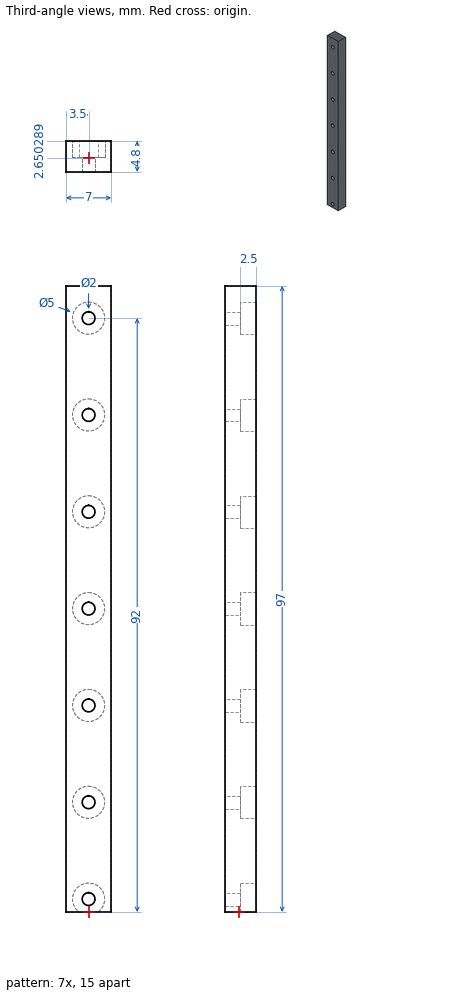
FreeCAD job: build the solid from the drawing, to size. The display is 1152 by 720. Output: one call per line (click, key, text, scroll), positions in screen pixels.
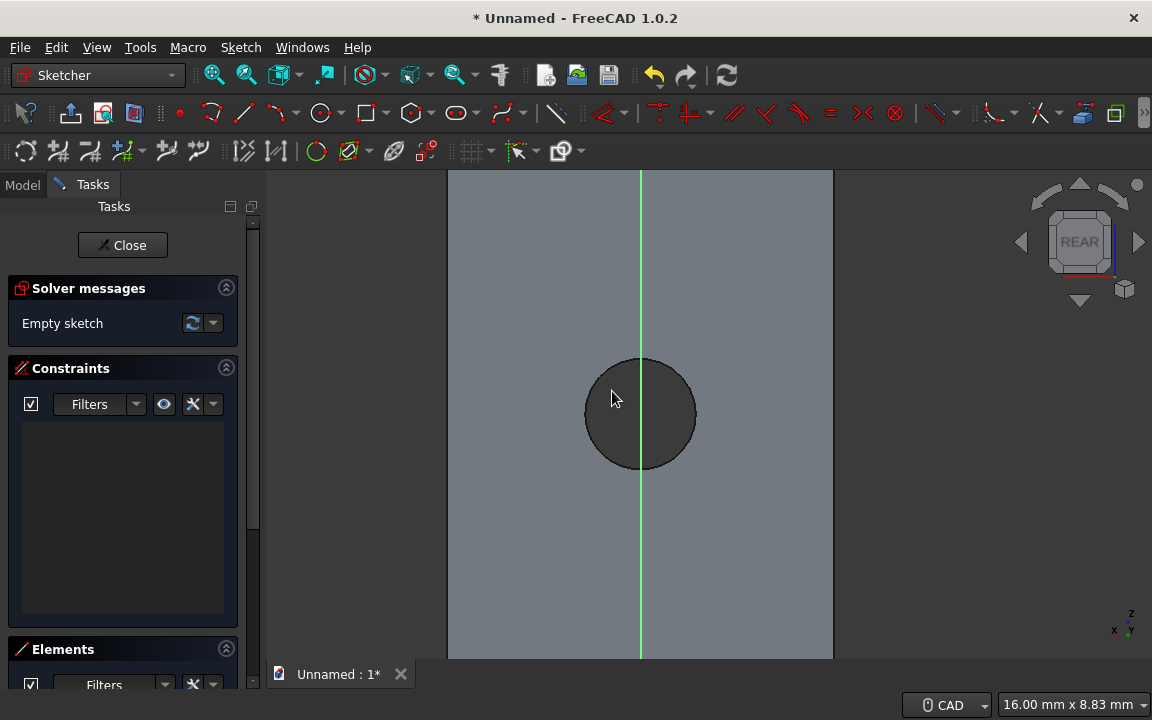
click(322, 114)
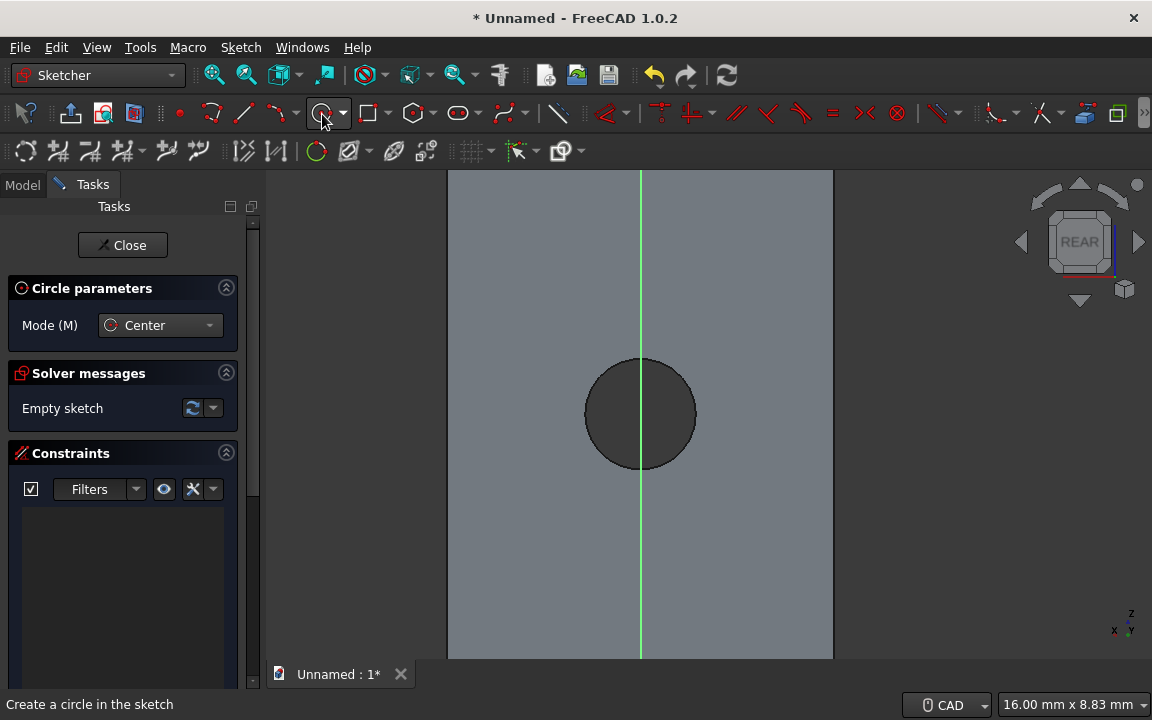
click(641, 414)
move(738, 316)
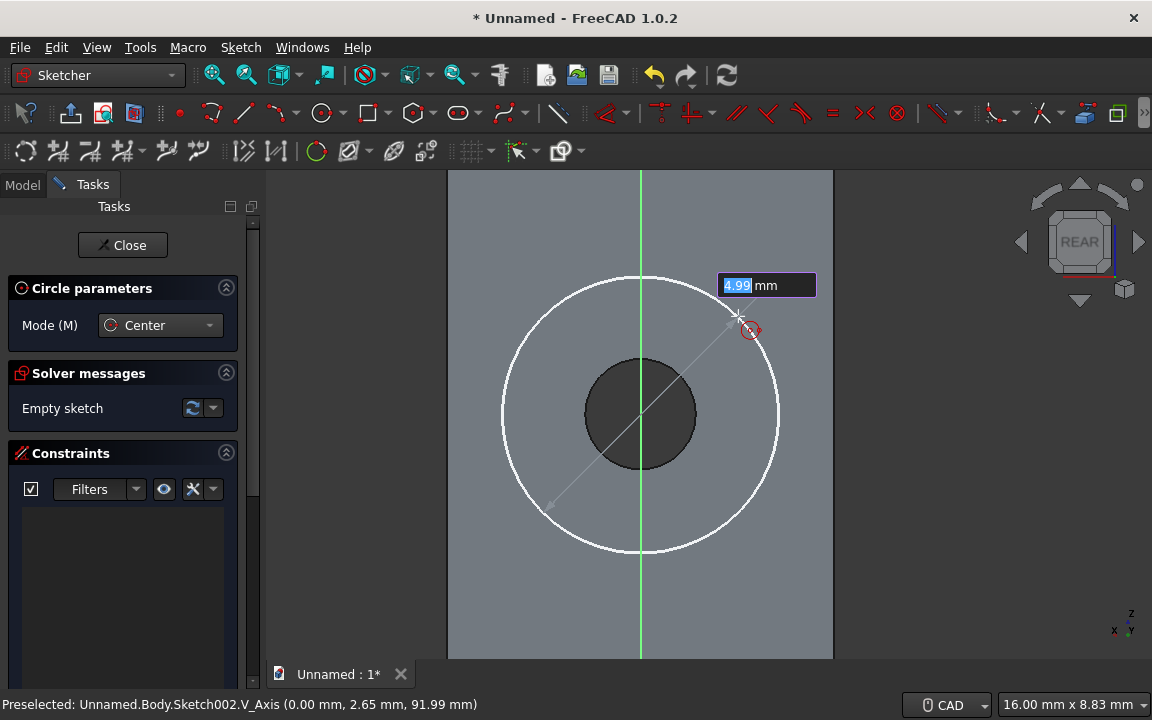
text(5)
key(Return)
key(Escape)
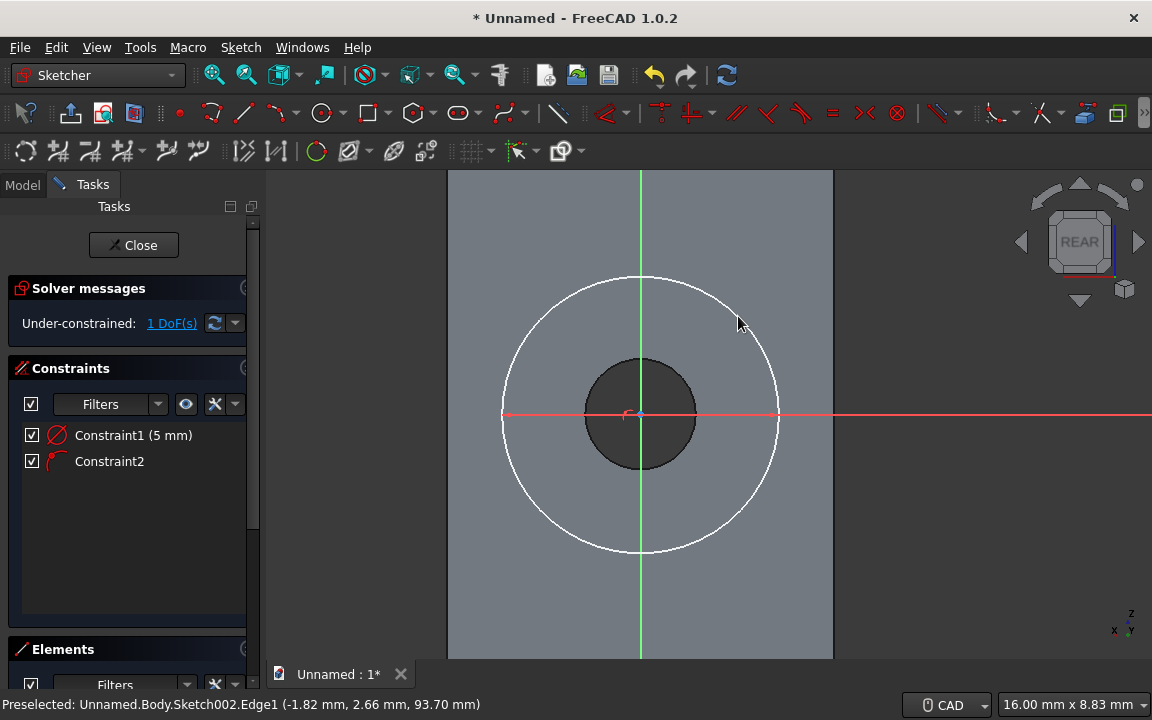
key(d)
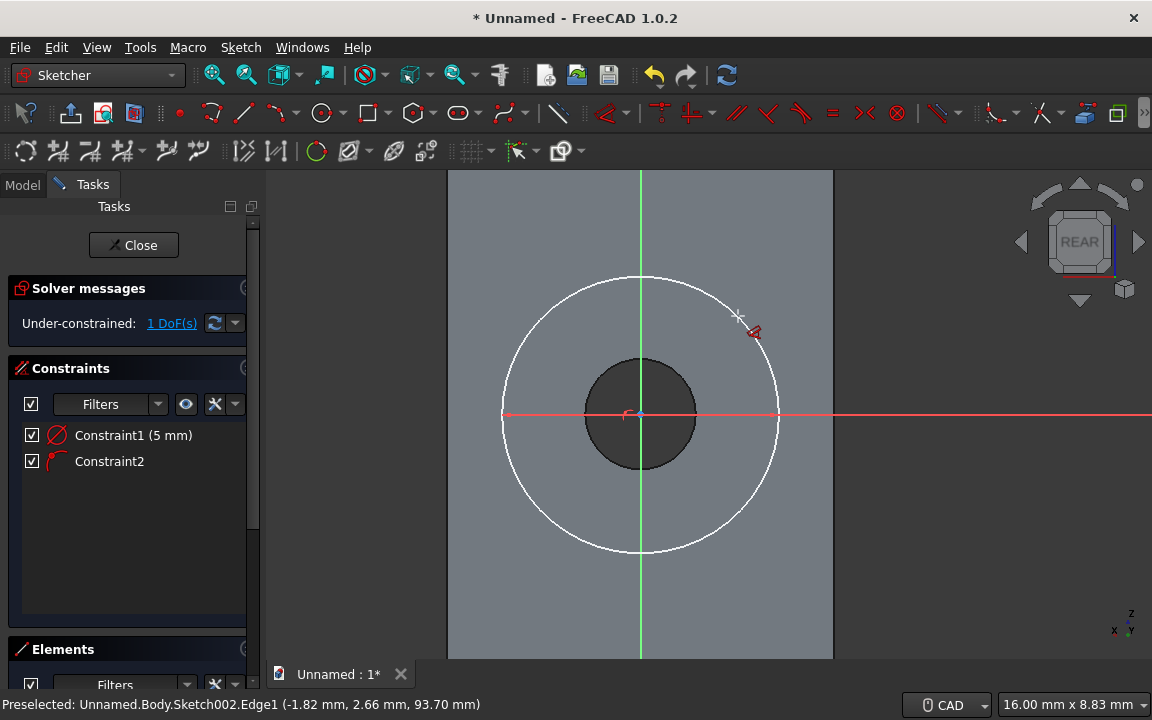
click(641, 415)
click(675, 523)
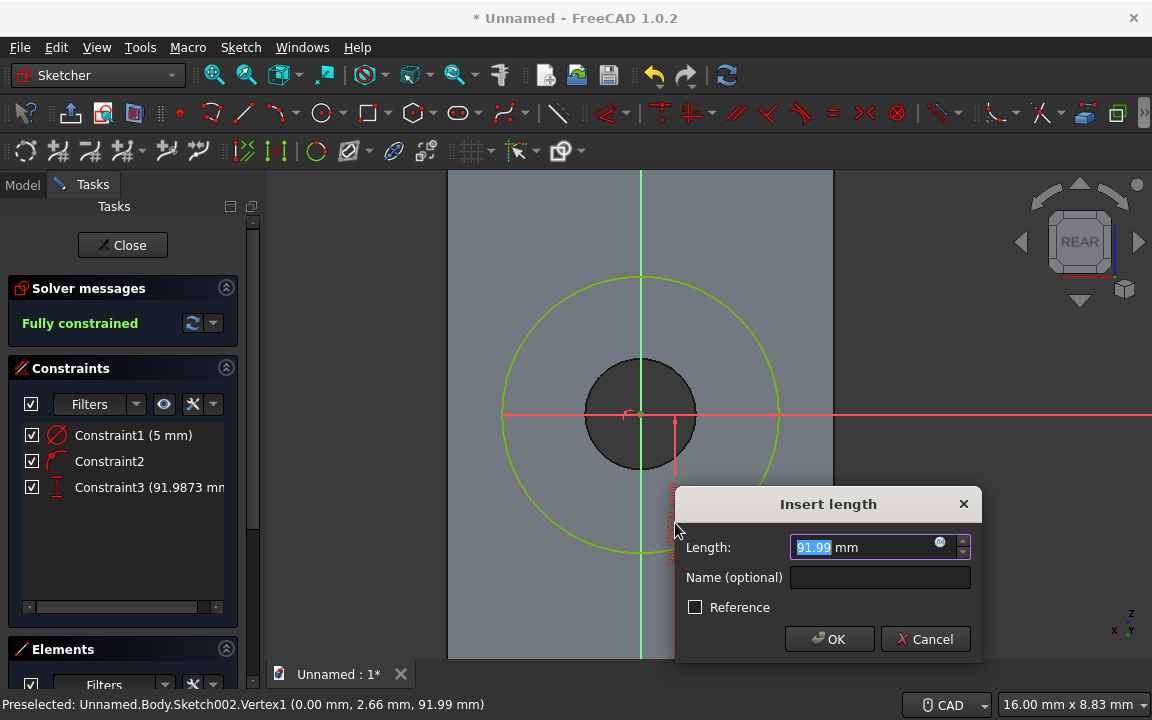
text(92)
key(Return)
key(Escape)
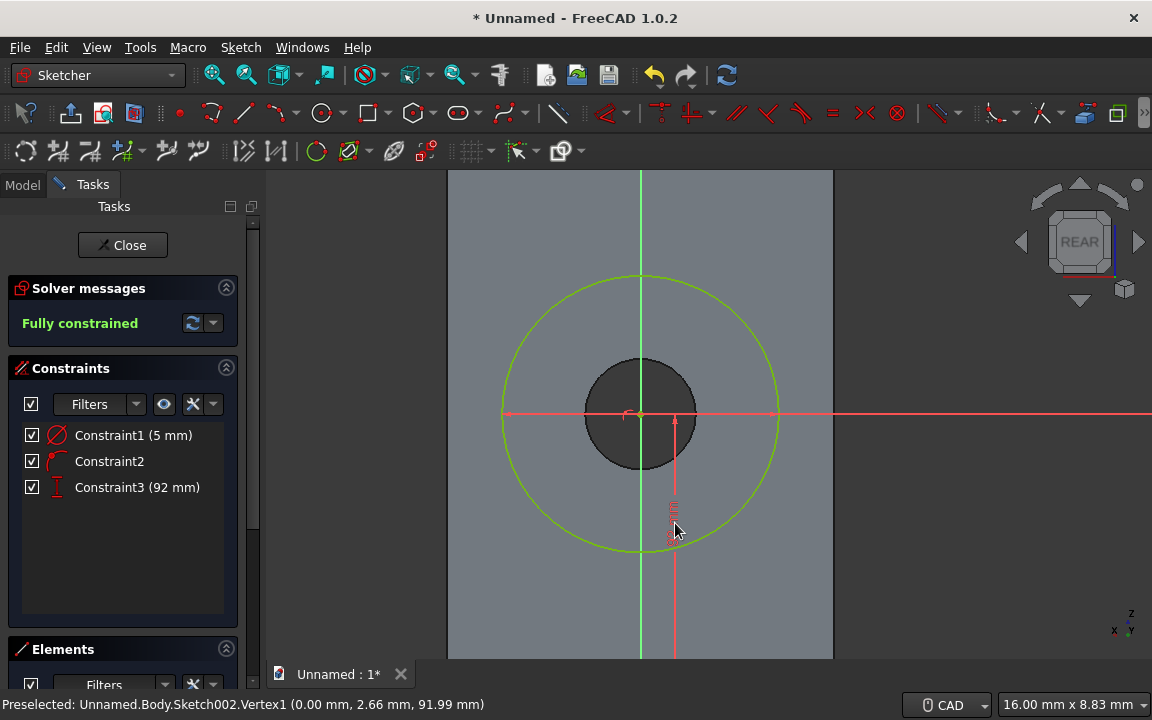
click(123, 245)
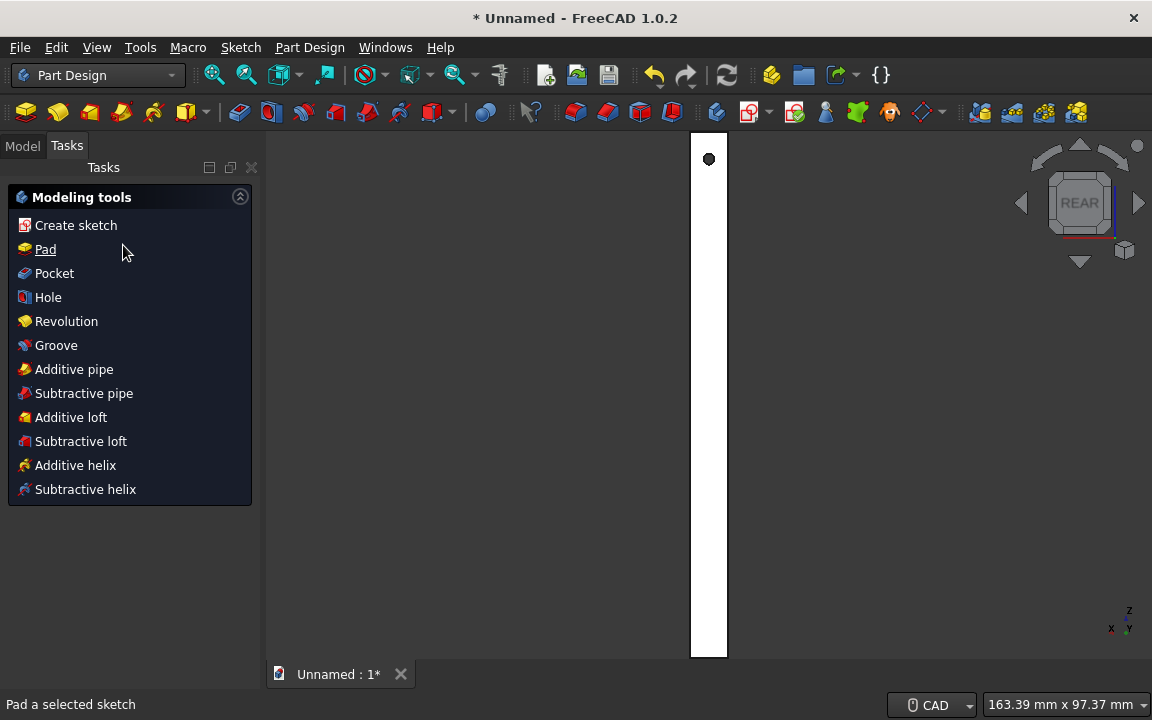
click(240, 112)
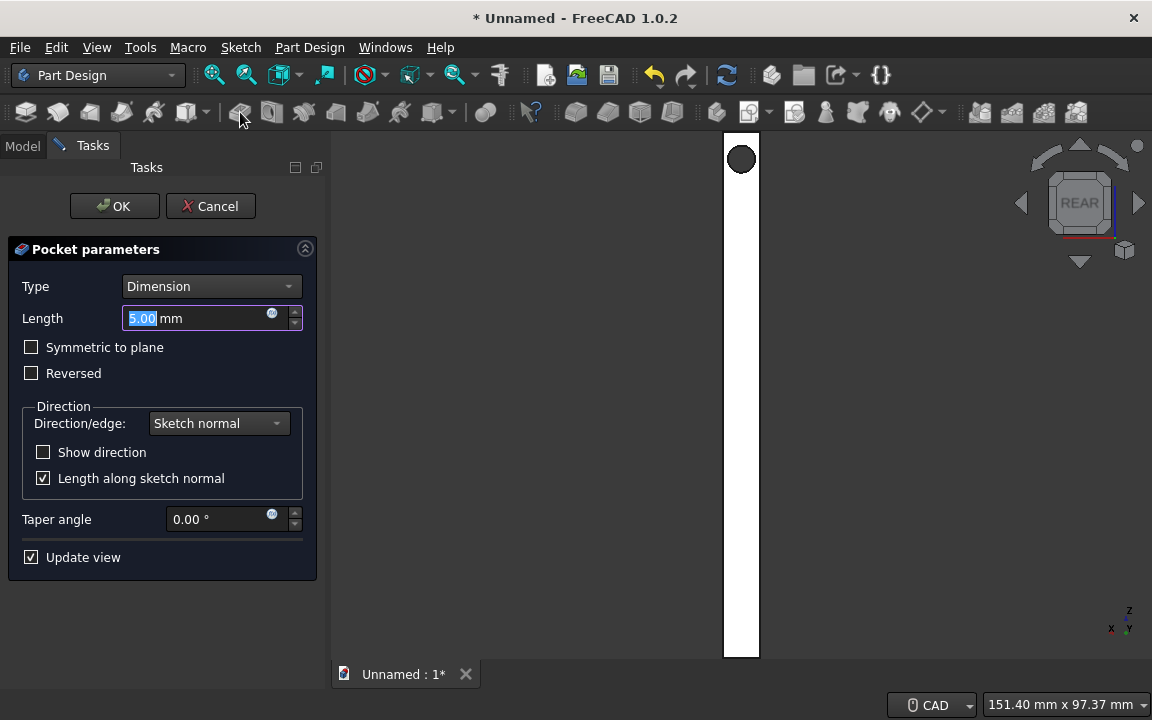
text(2.5)
key(Tab)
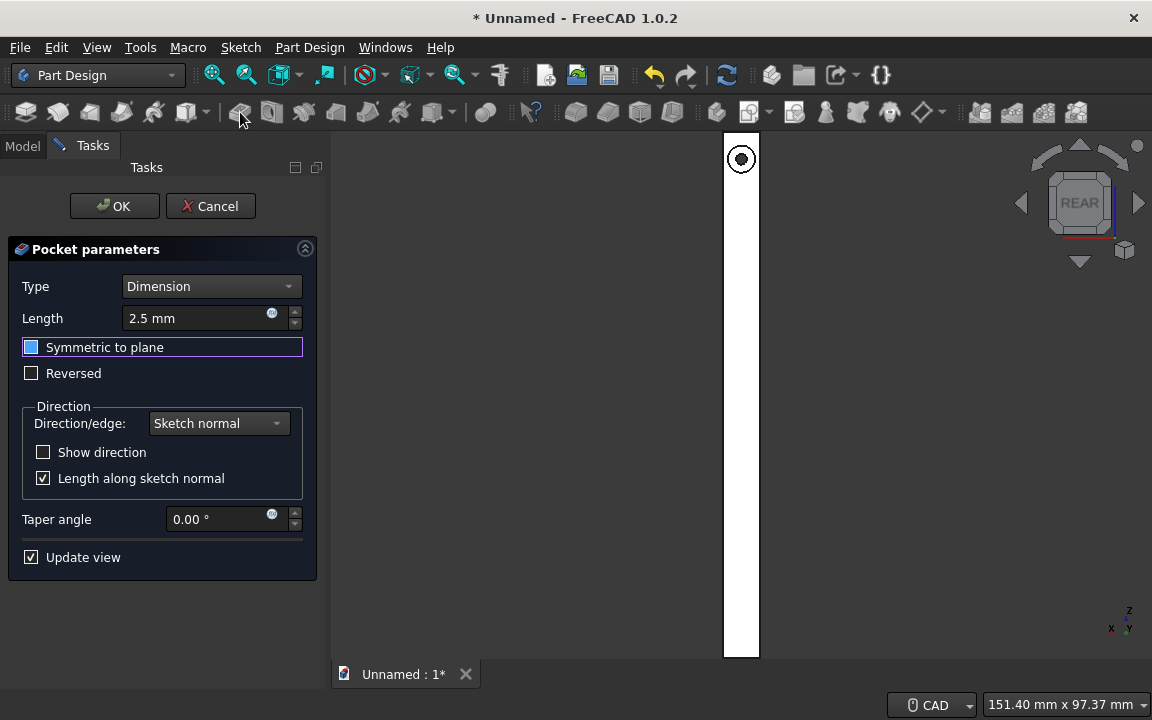
click(115, 206)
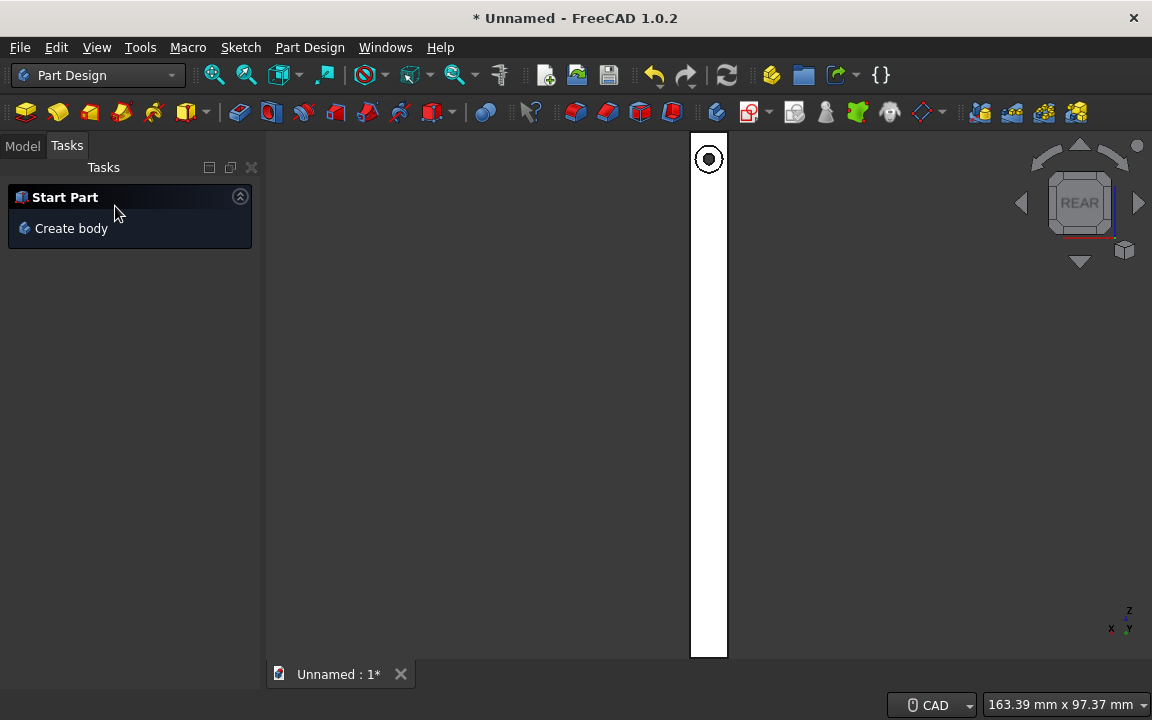
click(23, 145)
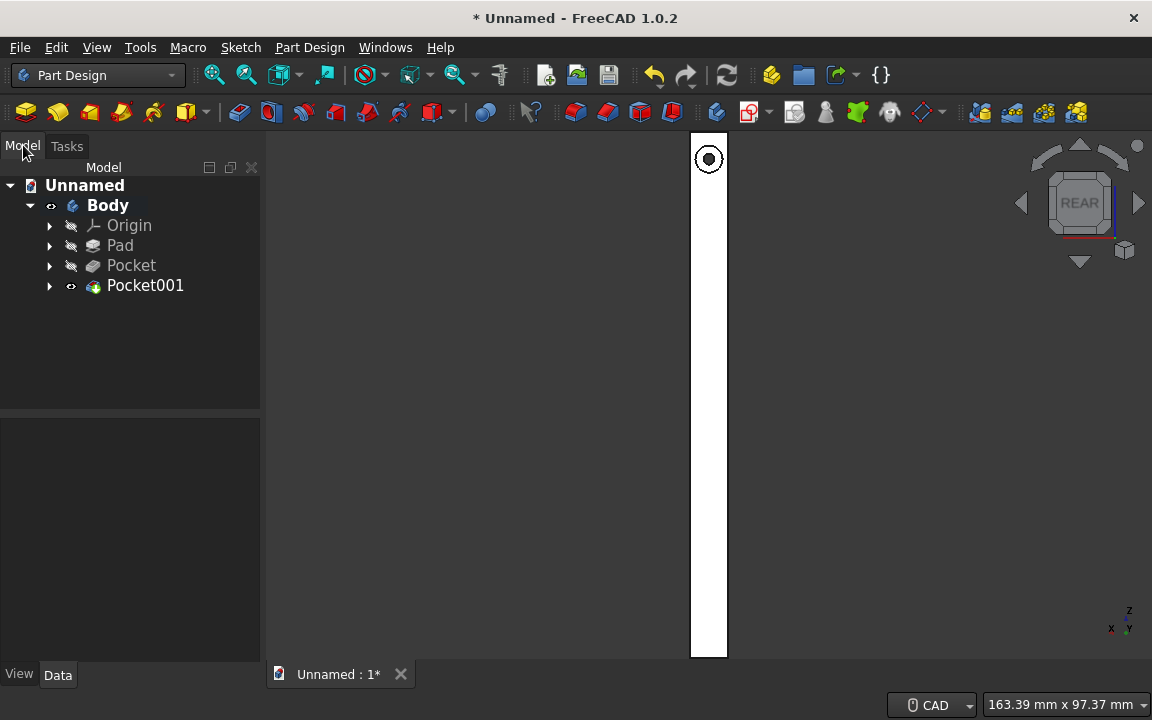
click(116, 266)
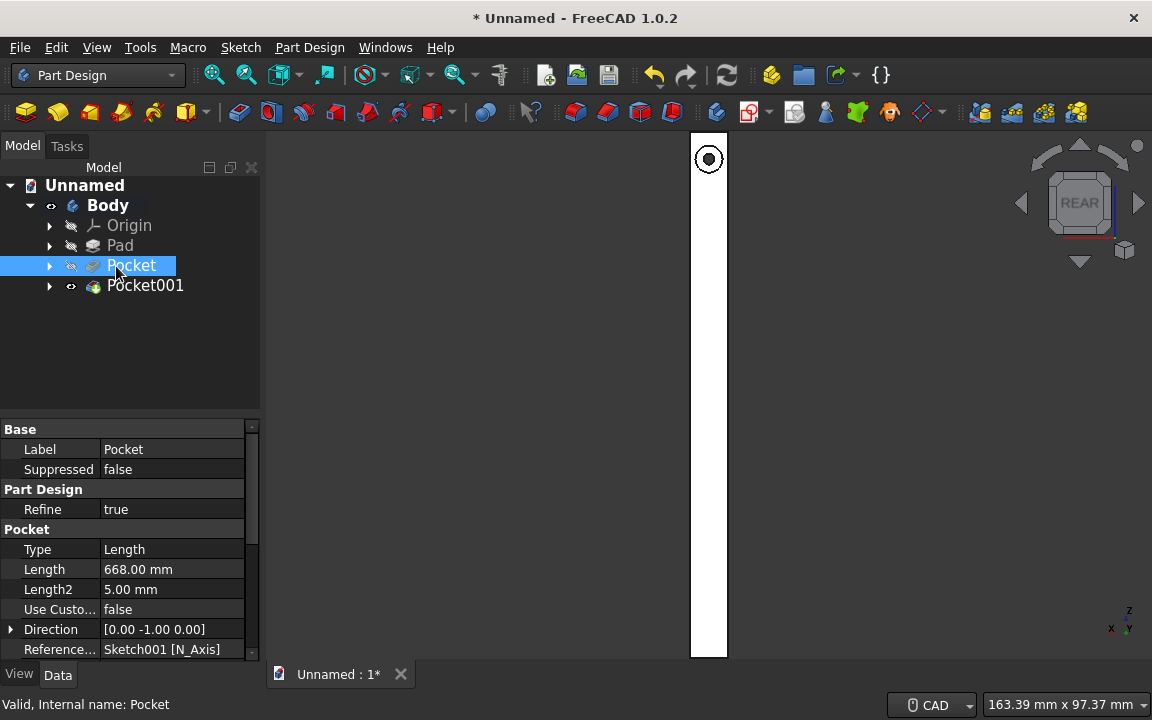
click(116, 286, ctrl)